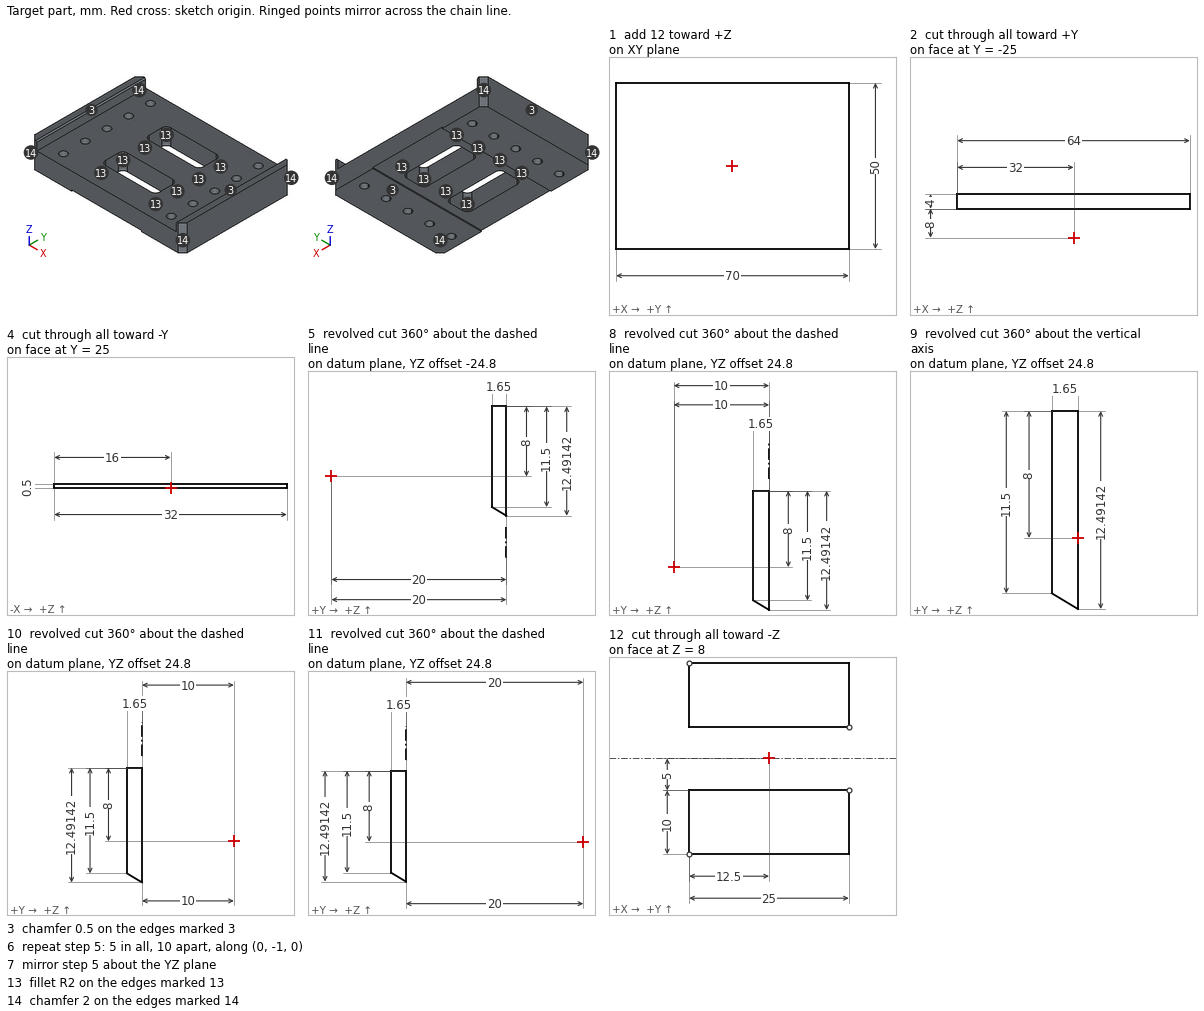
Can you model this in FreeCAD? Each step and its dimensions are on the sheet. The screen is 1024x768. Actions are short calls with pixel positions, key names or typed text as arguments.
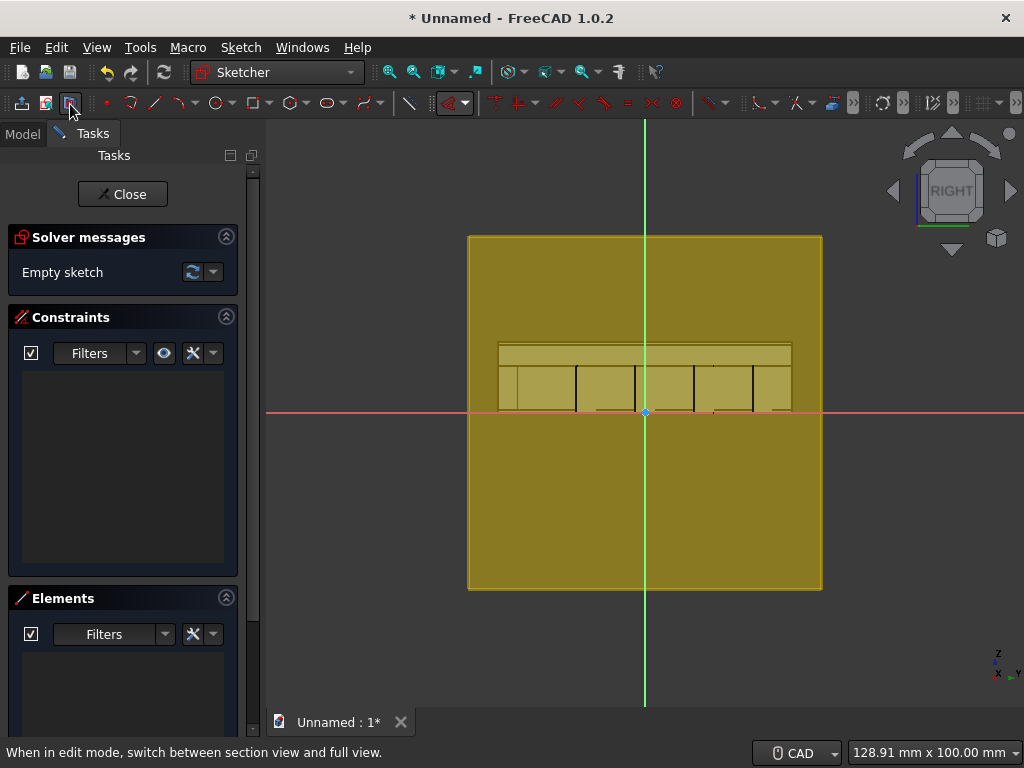
scroll(583, 377, up, 6)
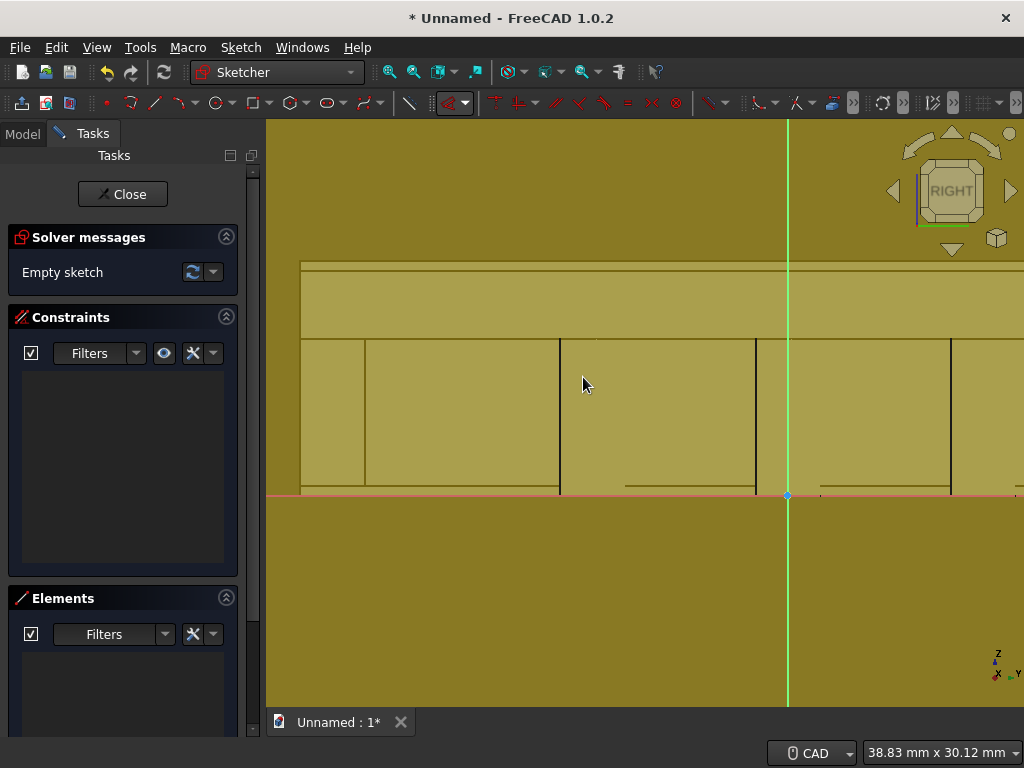
key(g)
key(m)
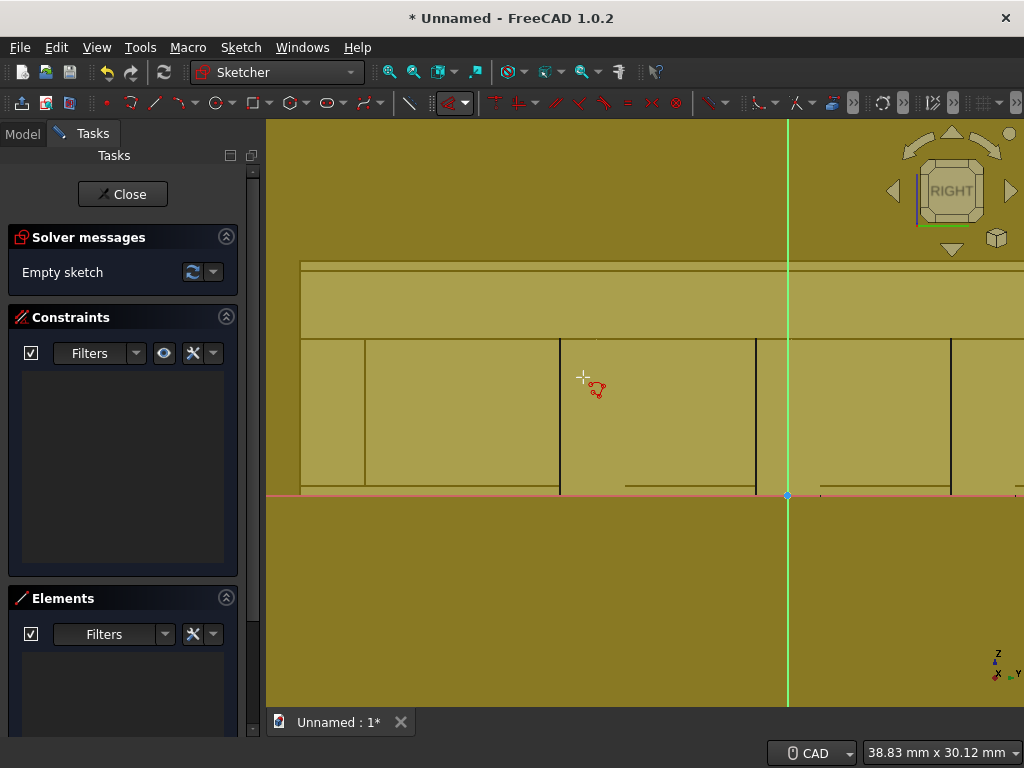
click(397, 583)
click(365, 564)
click(365, 339)
click(397, 339)
click(397, 584)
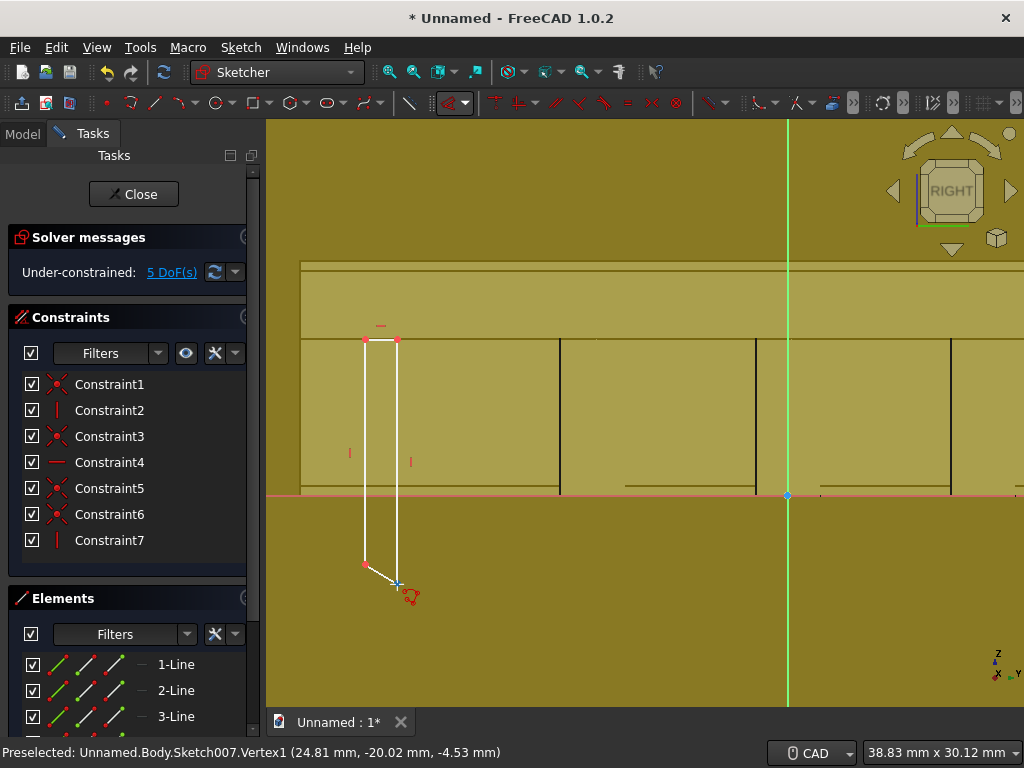
key(g)
key(l)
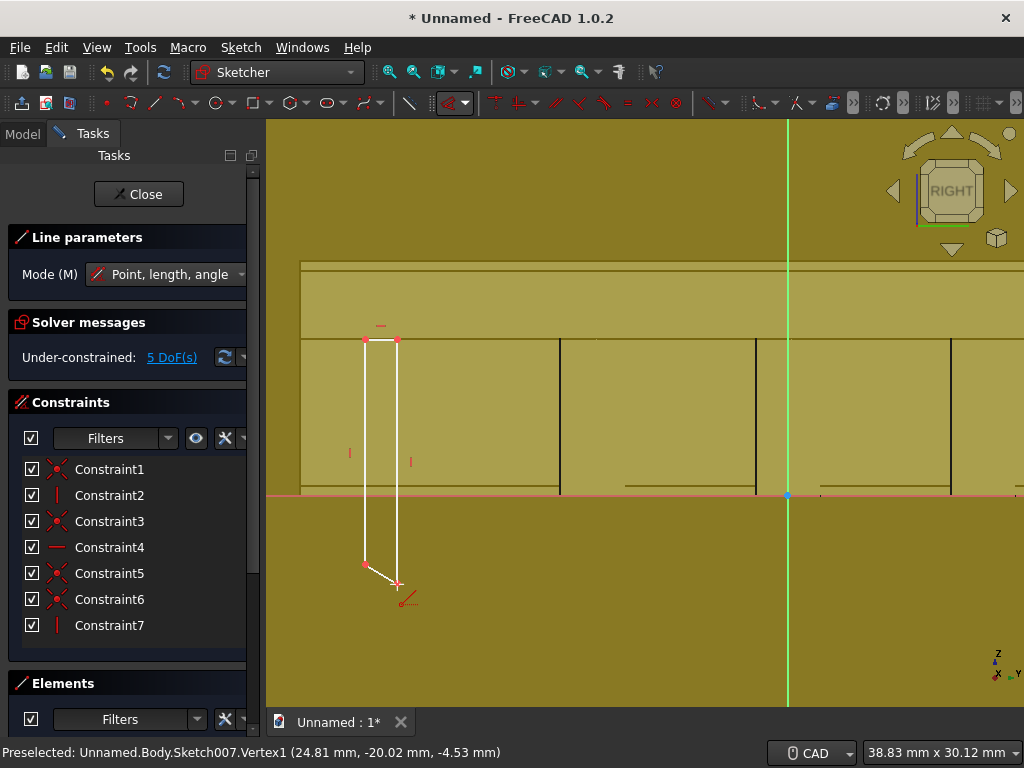
click(397, 315)
click(397, 242)
key(Escape)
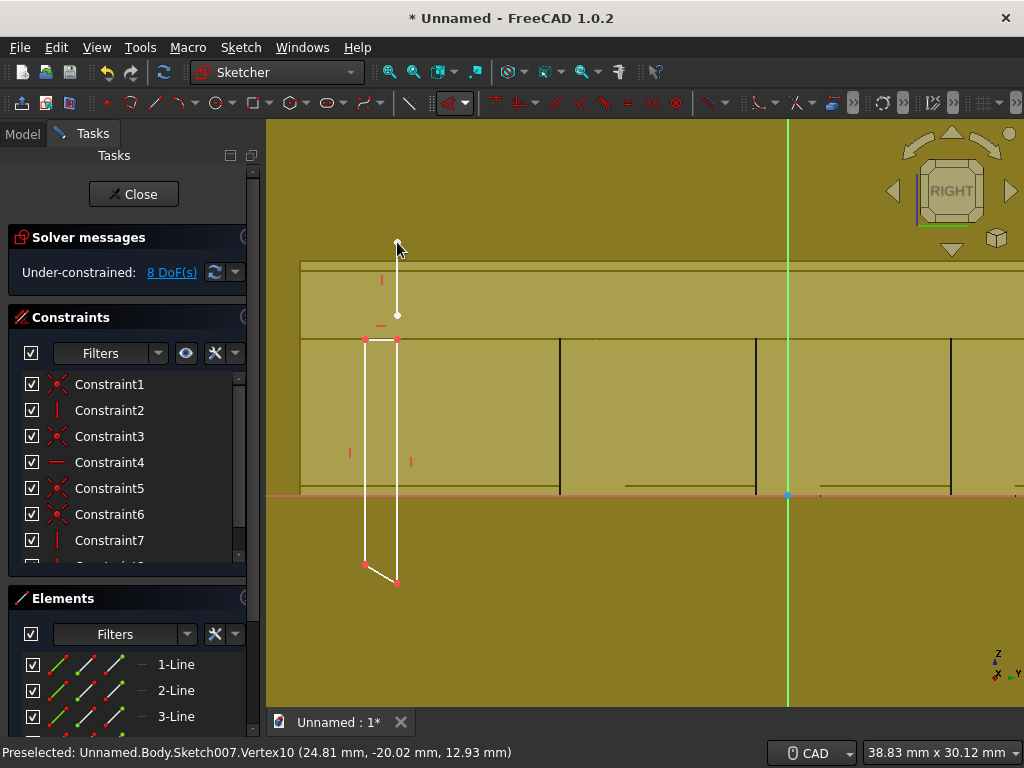
click(397, 294)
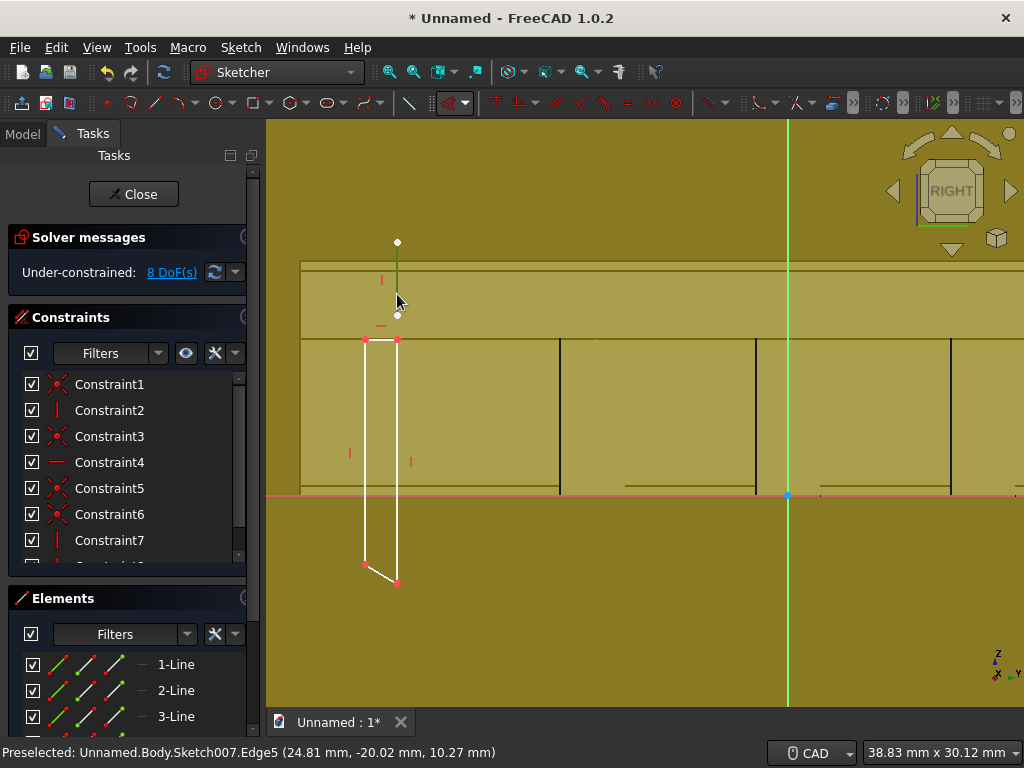
key(g)
key(n)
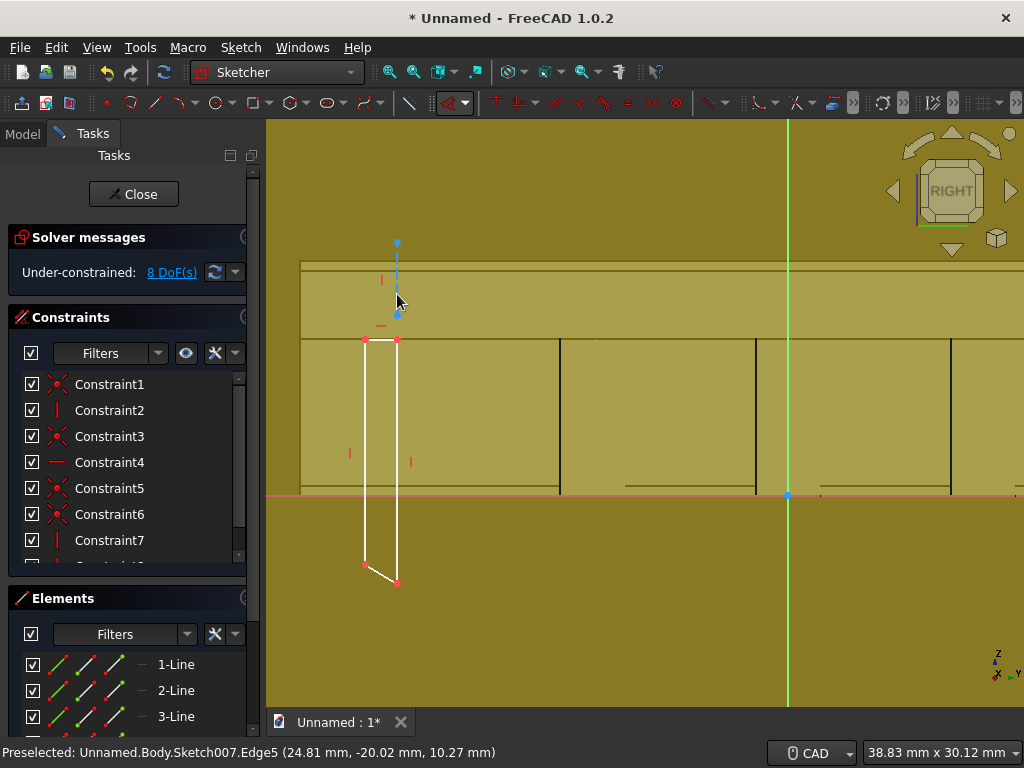
click(365, 340)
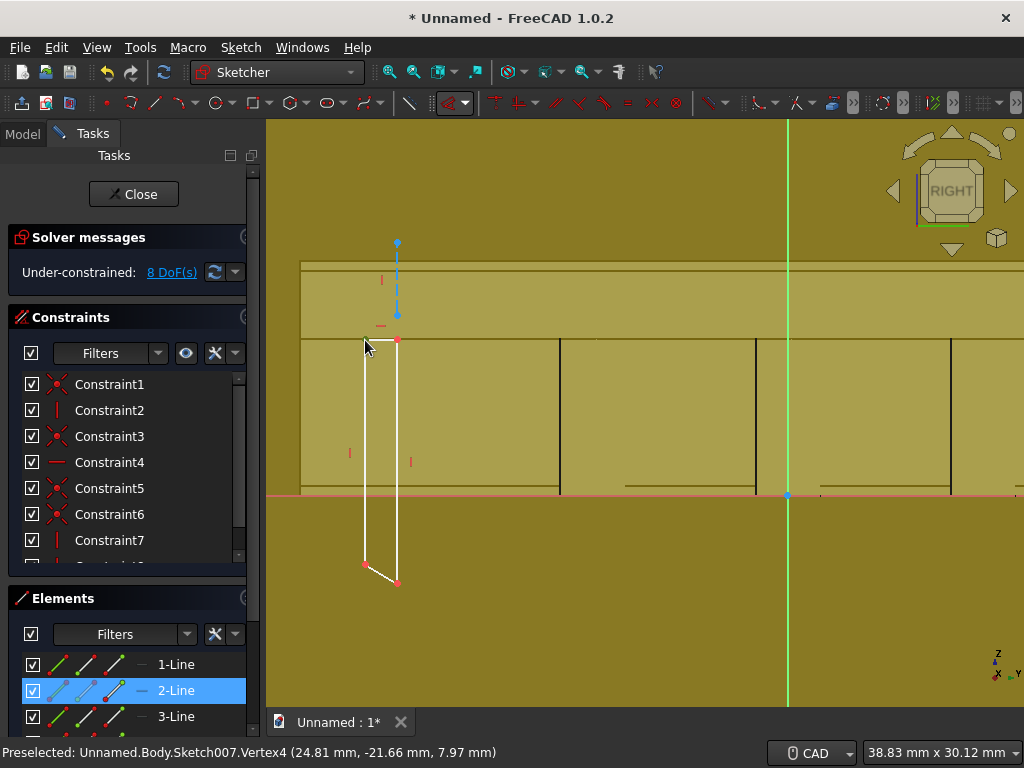
click(468, 104)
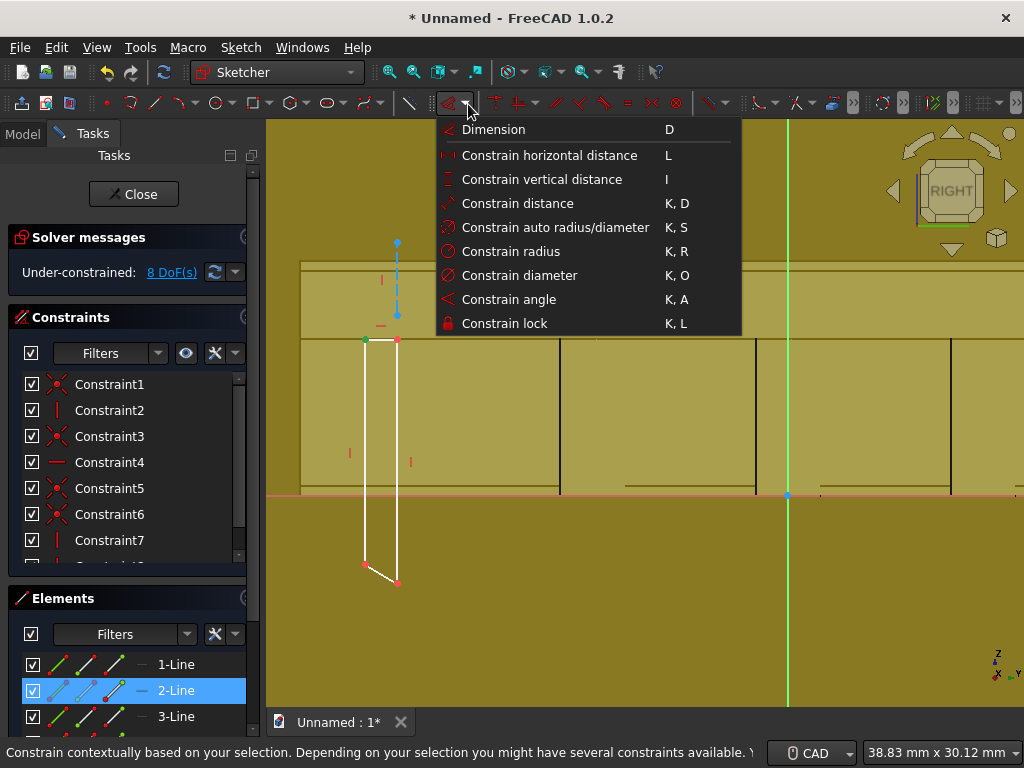
click(589, 179)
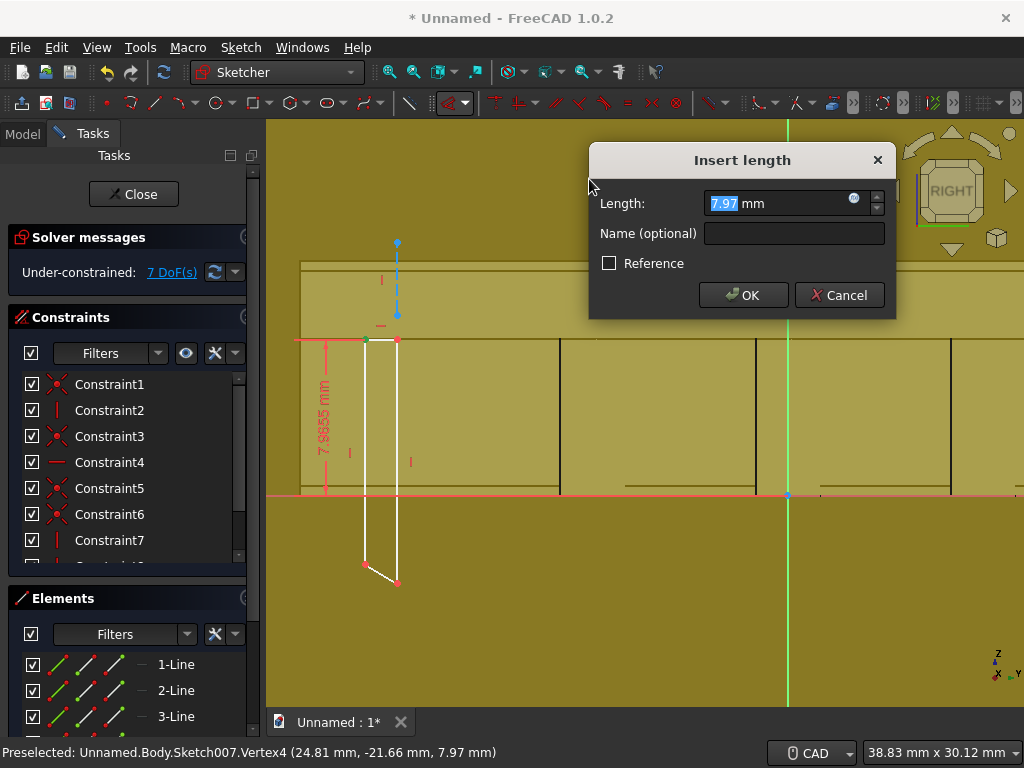
text(8)
key(Return)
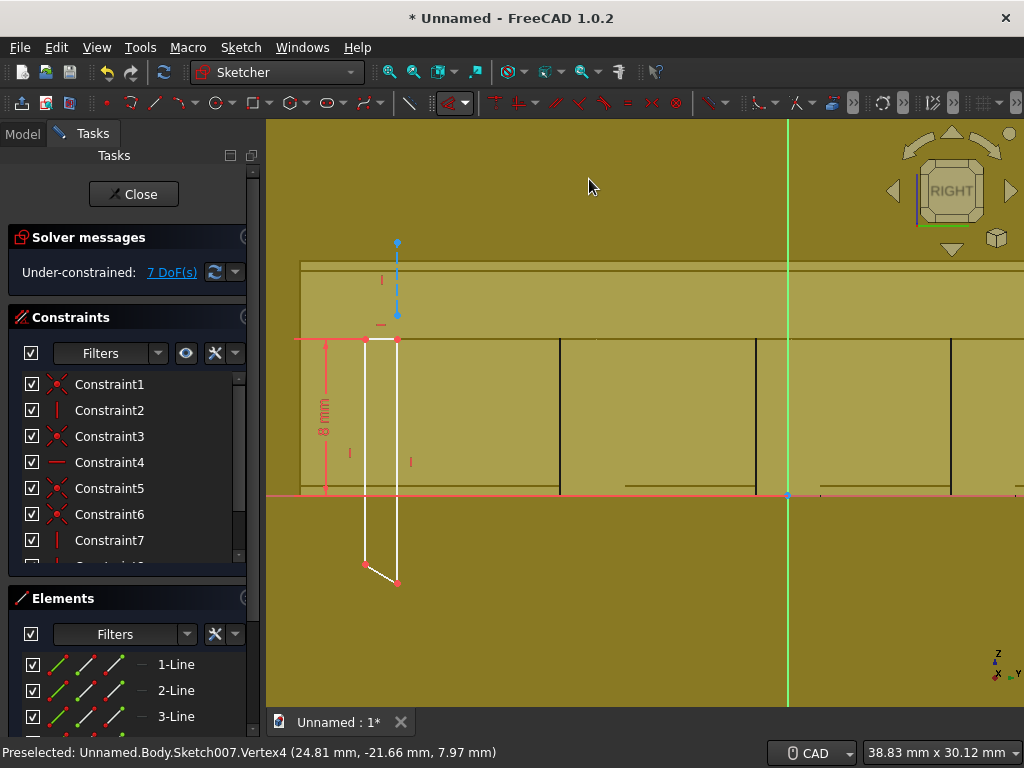
click(397, 584)